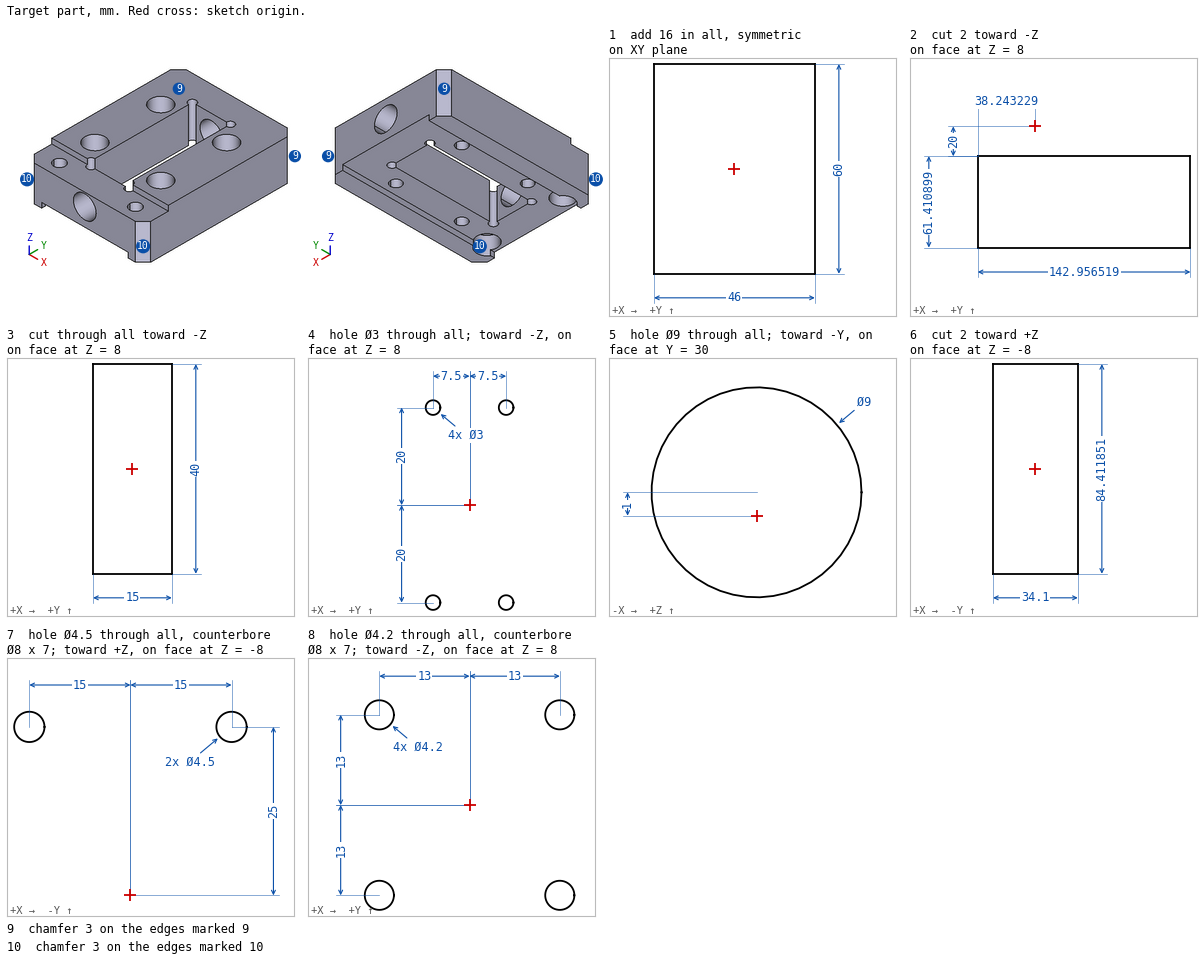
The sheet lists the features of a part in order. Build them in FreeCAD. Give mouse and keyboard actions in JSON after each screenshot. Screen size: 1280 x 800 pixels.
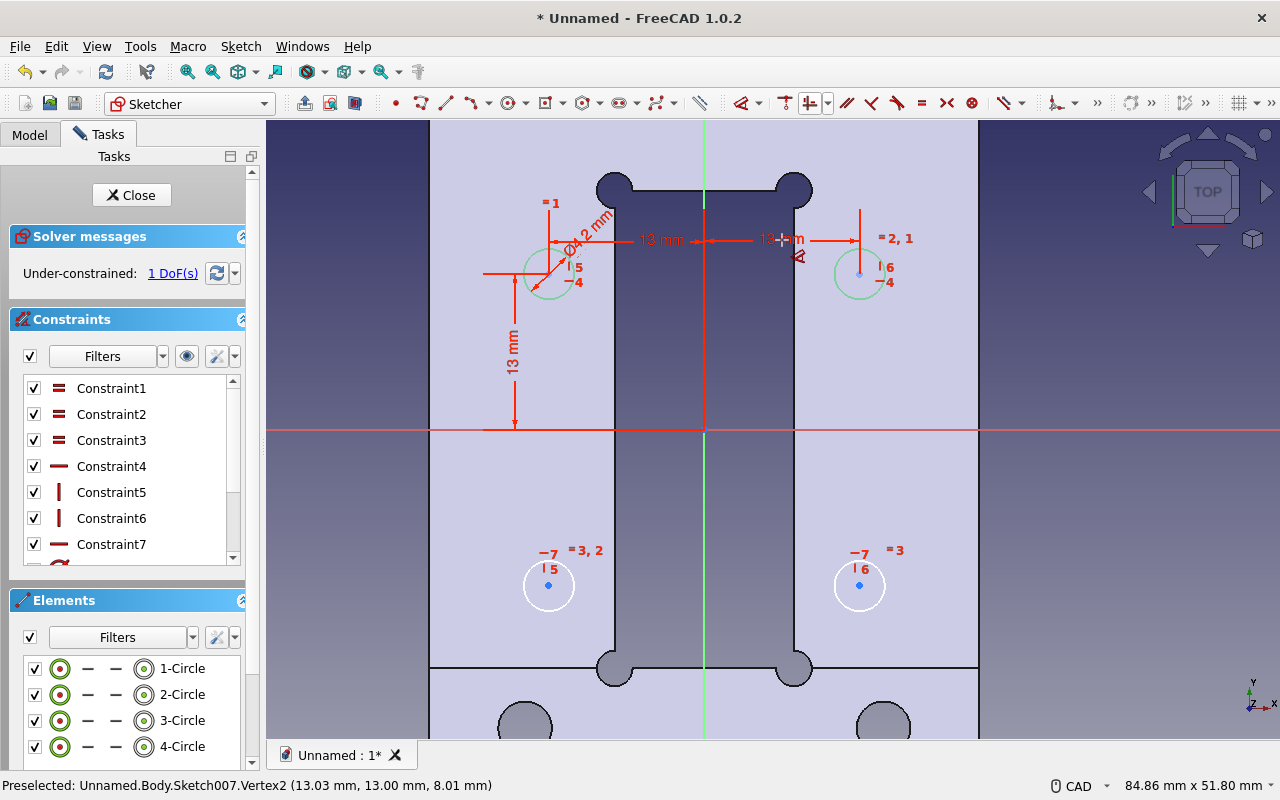
{"action": "left_click", "coordinate": [549, 586]}
{"action": "left_click", "coordinate": [515, 508]}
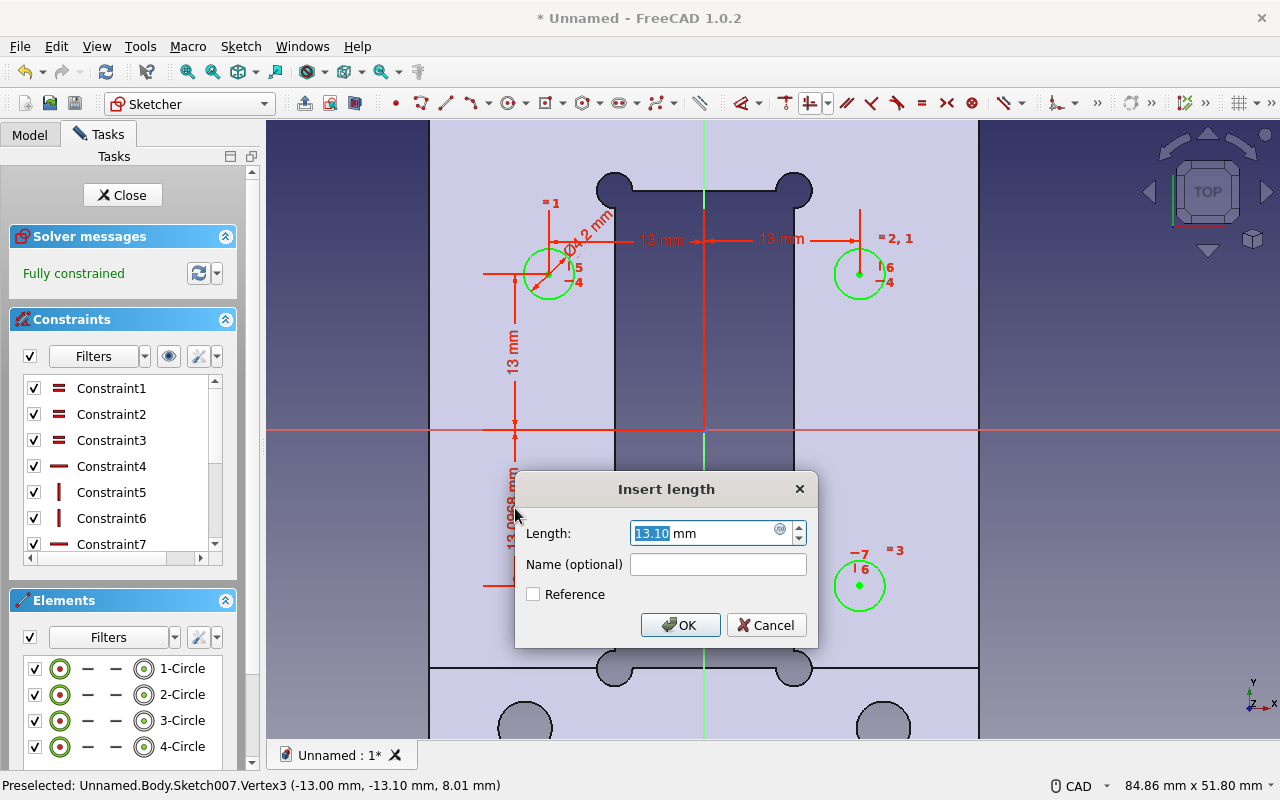
{"action": "type", "text": "13"}
{"action": "key", "text": "Return"}
{"action": "key", "text": "Escape"}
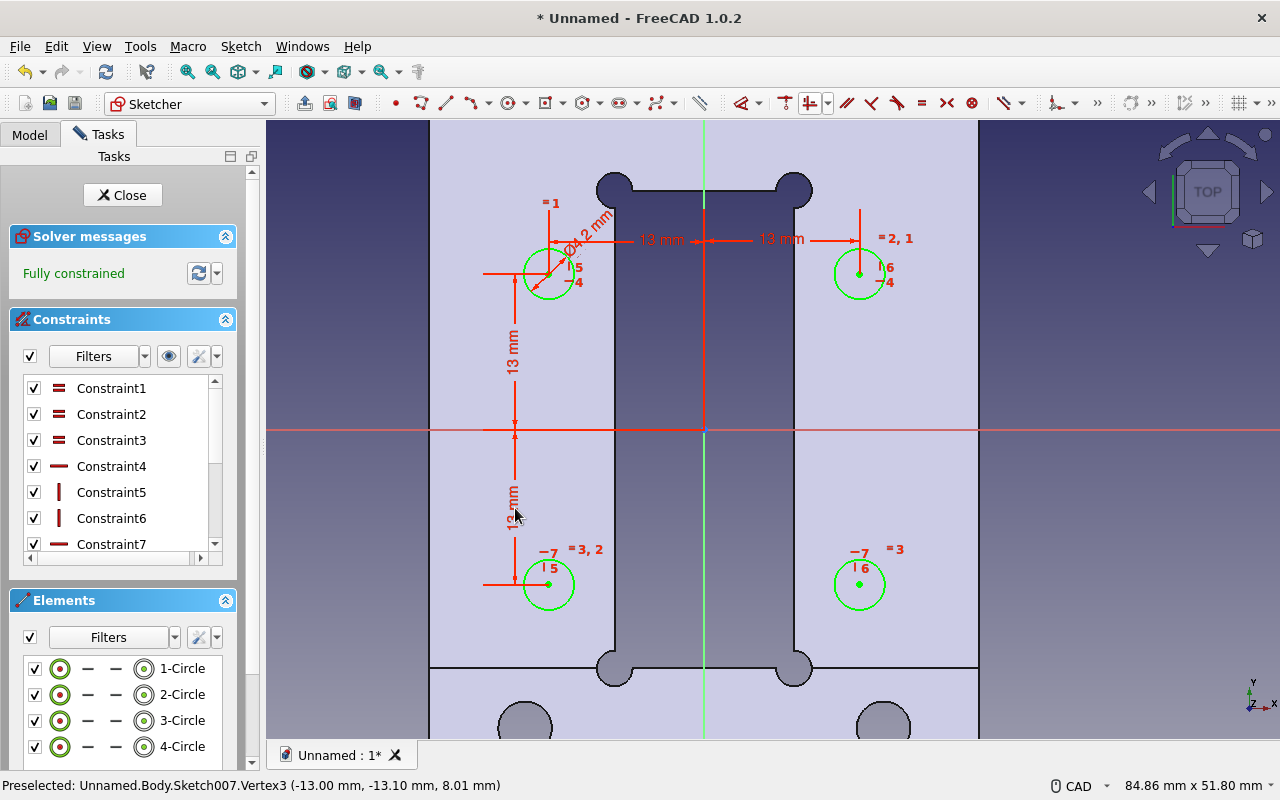
{"action": "left_click", "coordinate": [123, 195]}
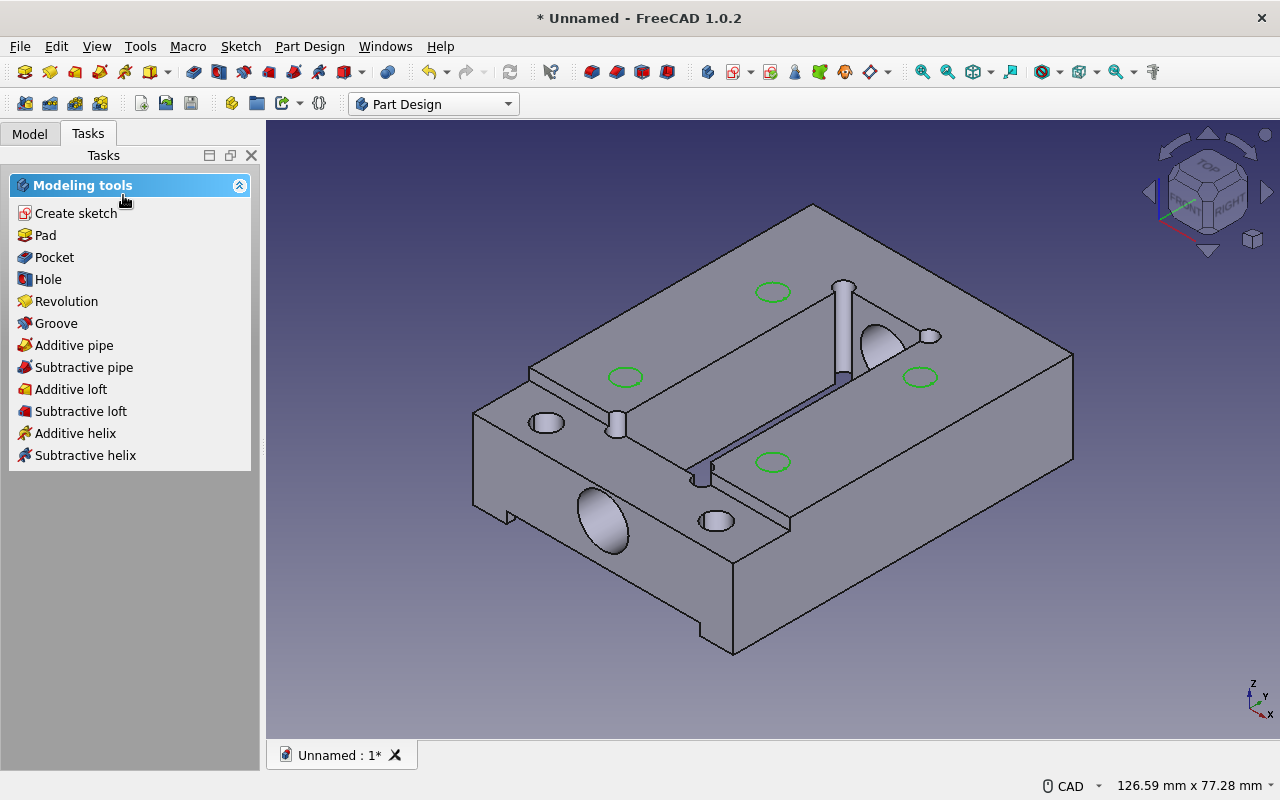
{"action": "left_click", "coordinate": [219, 72]}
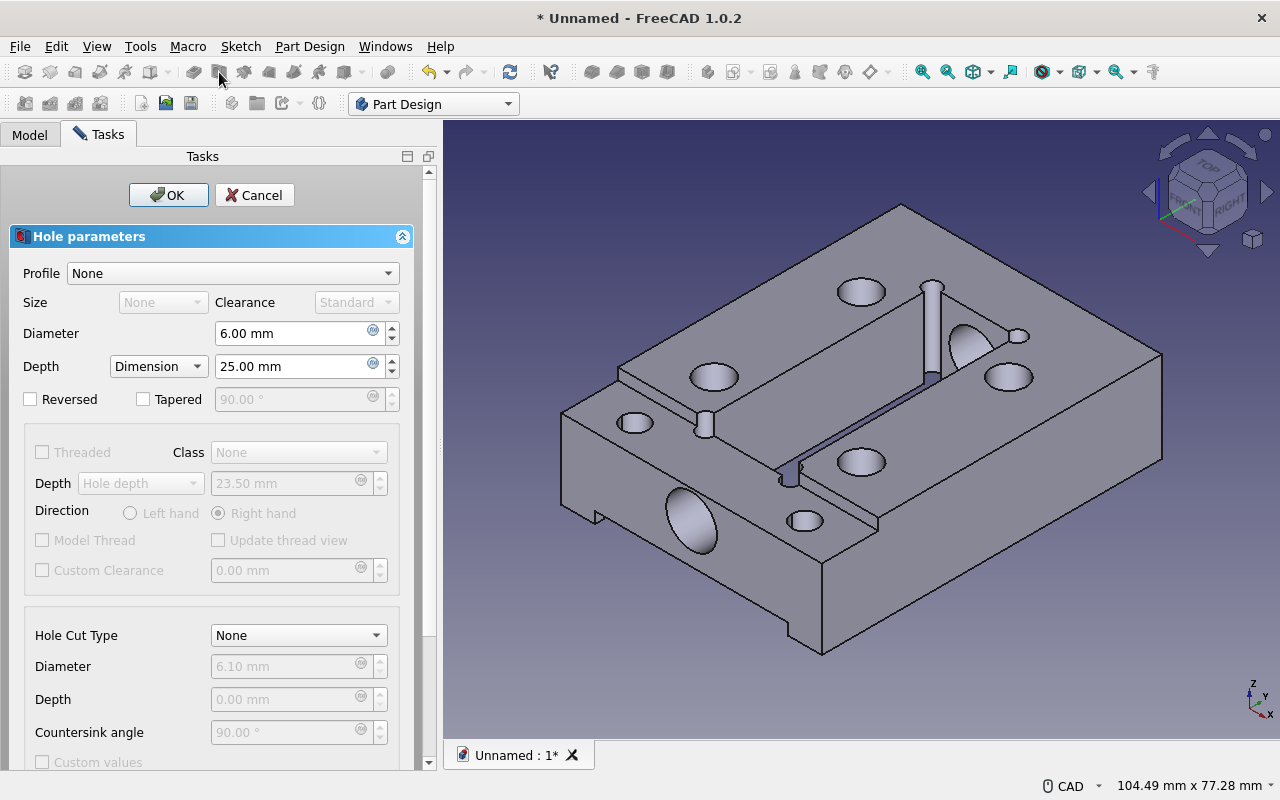
{"action": "triple_click", "coordinate": [300, 334]}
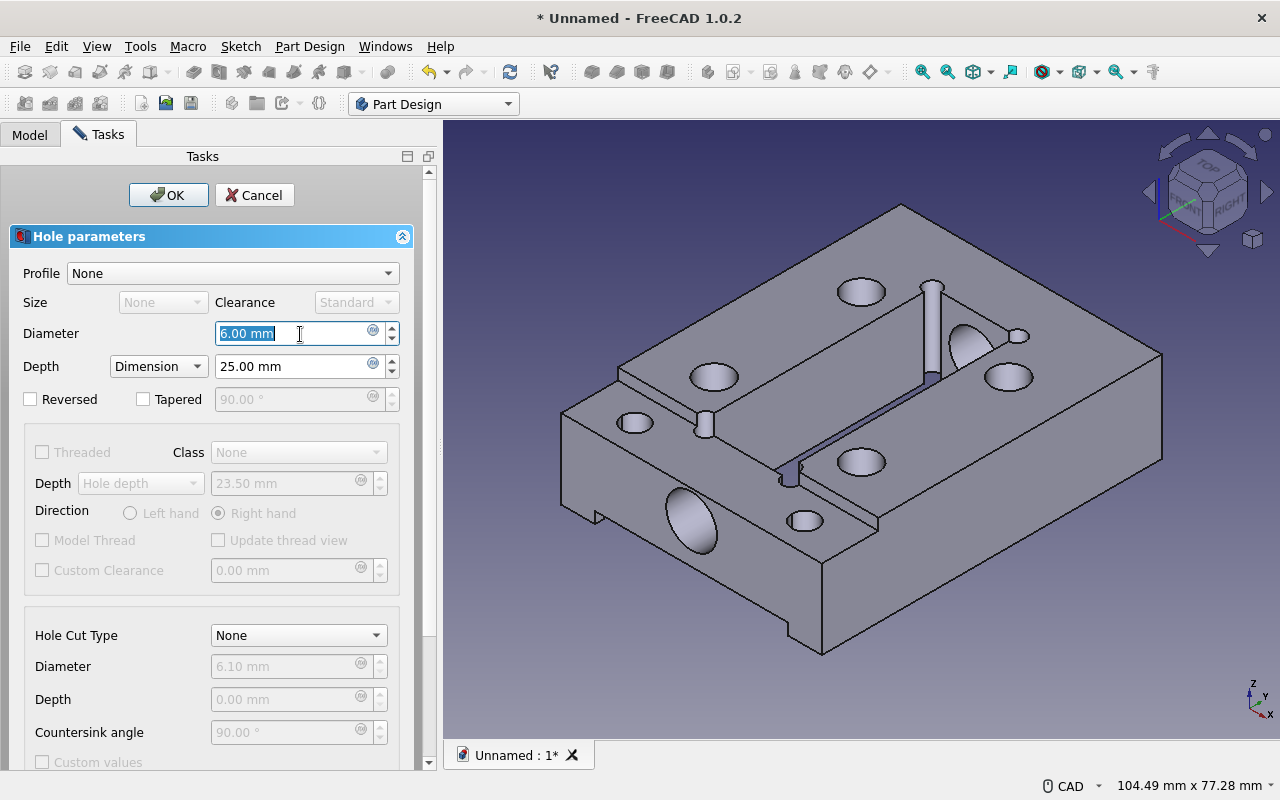
{"action": "type", "text": "4.2"}
{"action": "key", "text": "Tab"}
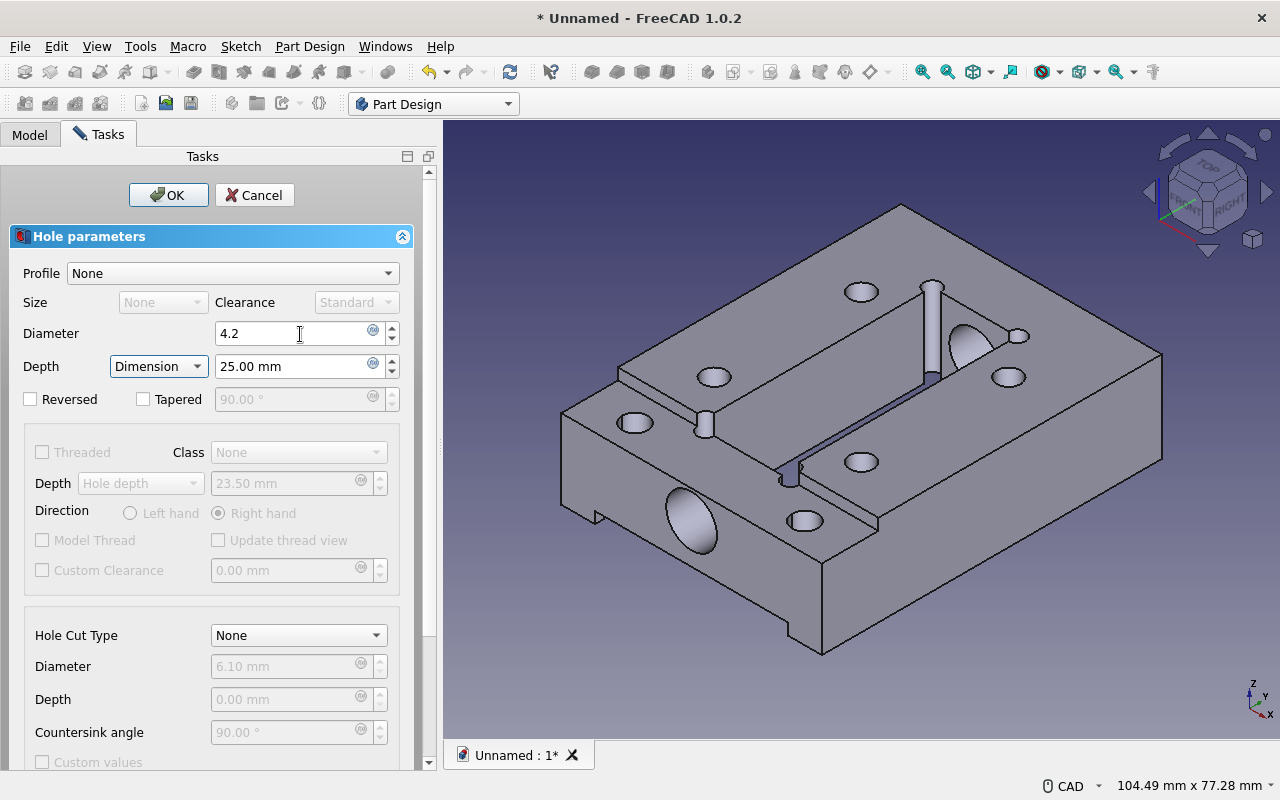
{"action": "left_click", "coordinate": [160, 366]}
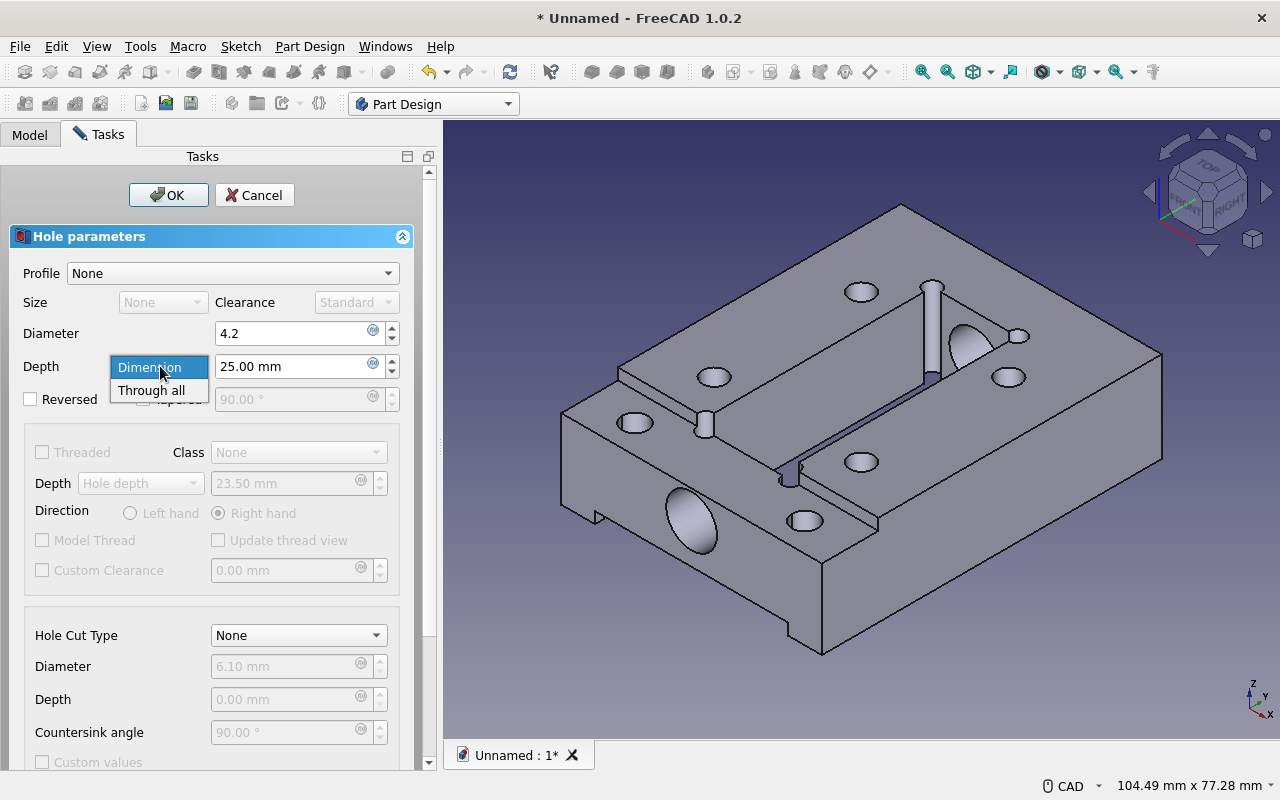
{"action": "left_click", "coordinate": [158, 390]}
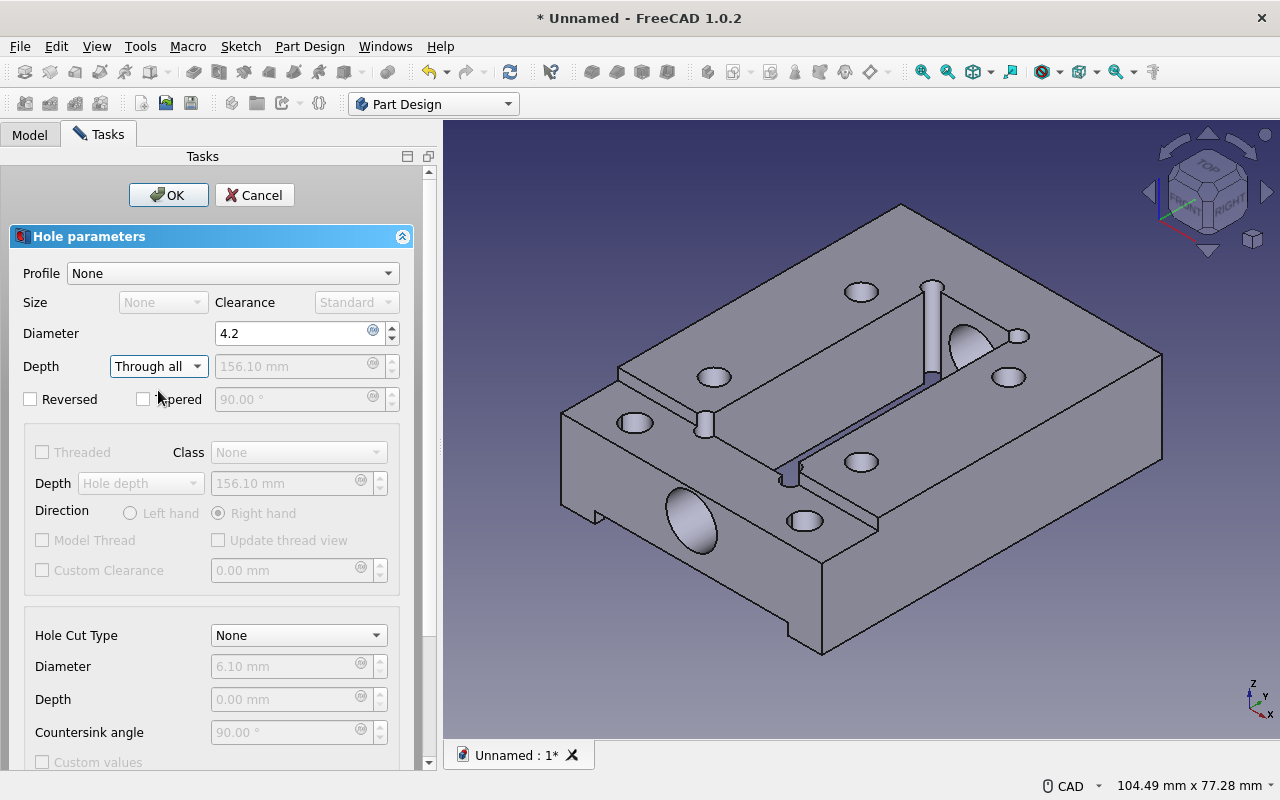
{"action": "left_click", "coordinate": [300, 636]}